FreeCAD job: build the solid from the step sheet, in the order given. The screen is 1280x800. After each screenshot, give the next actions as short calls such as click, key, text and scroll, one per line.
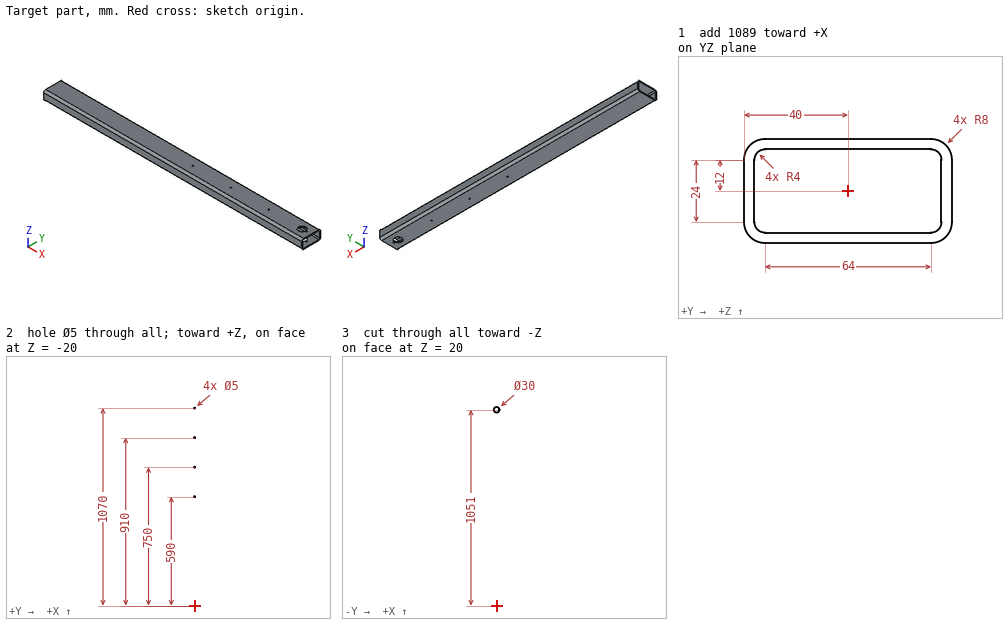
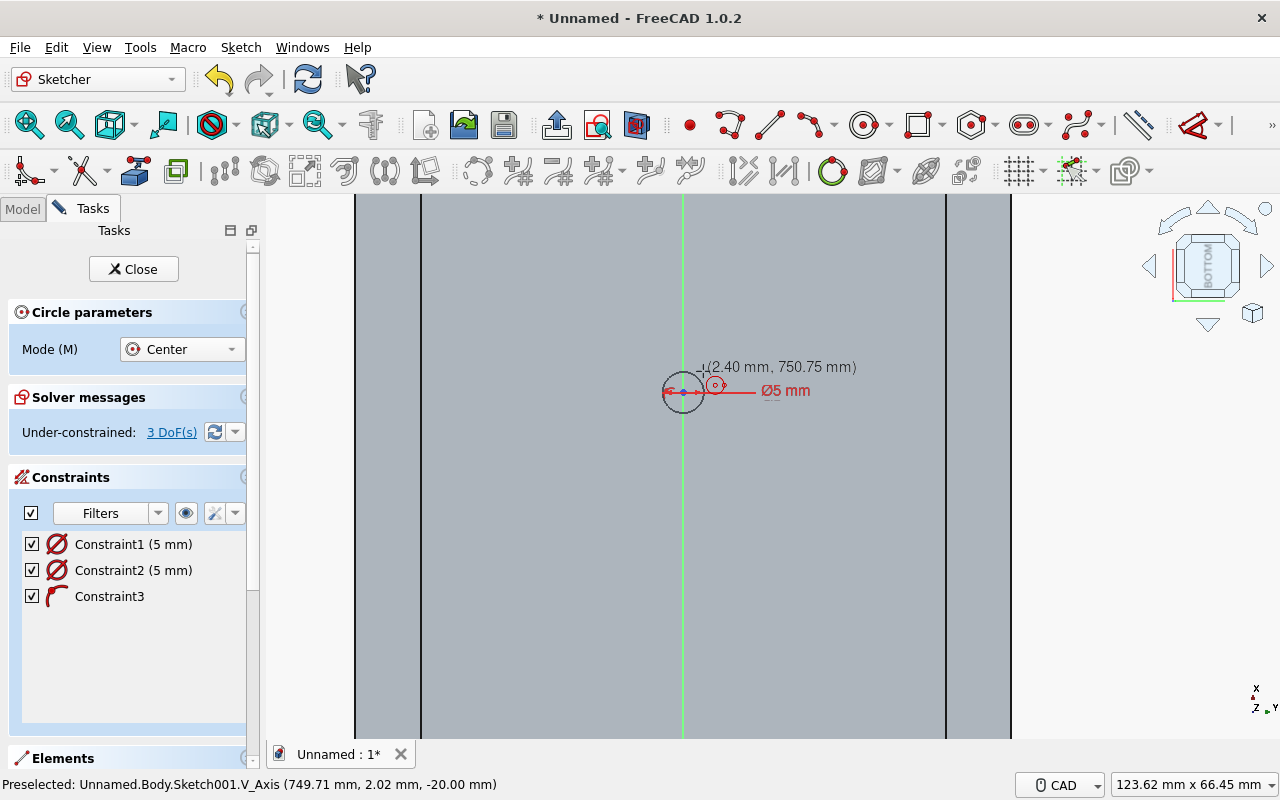
scroll(706, 379, down, 15)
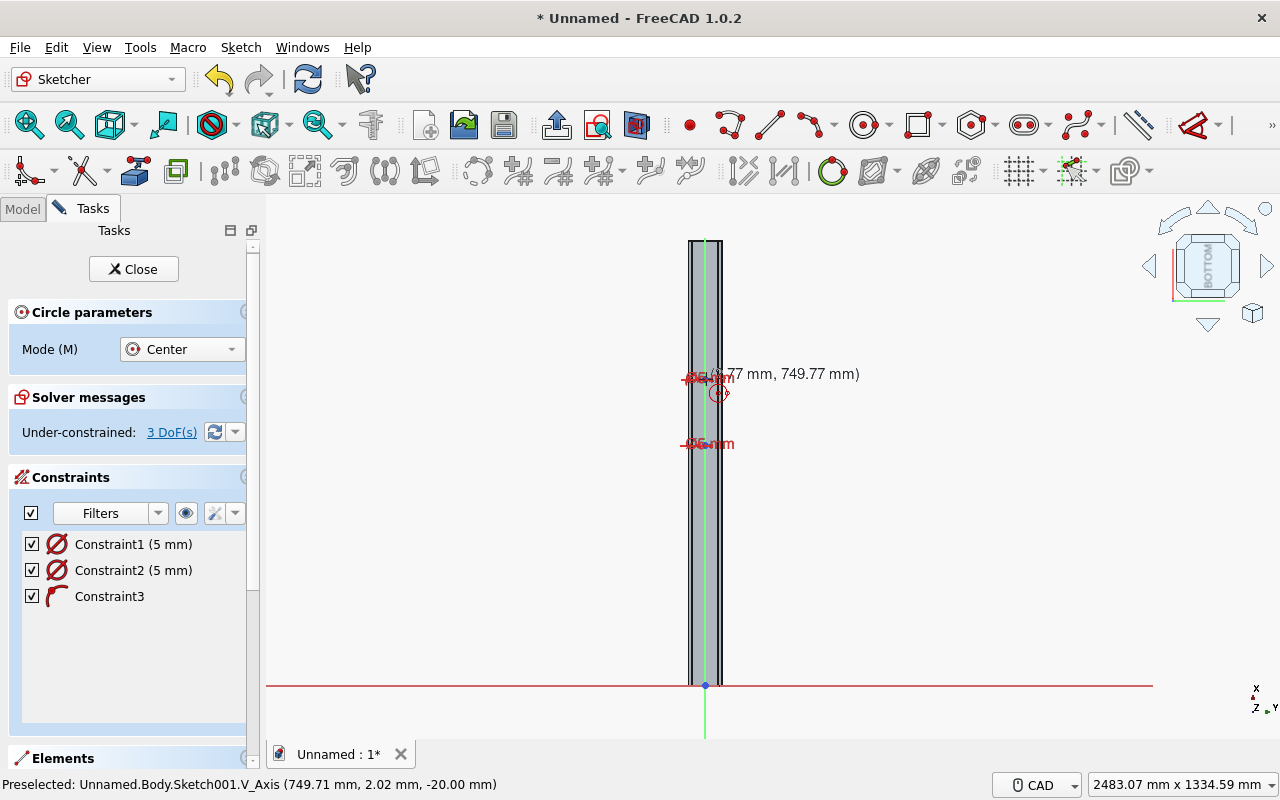
scroll(705, 314, up, 16)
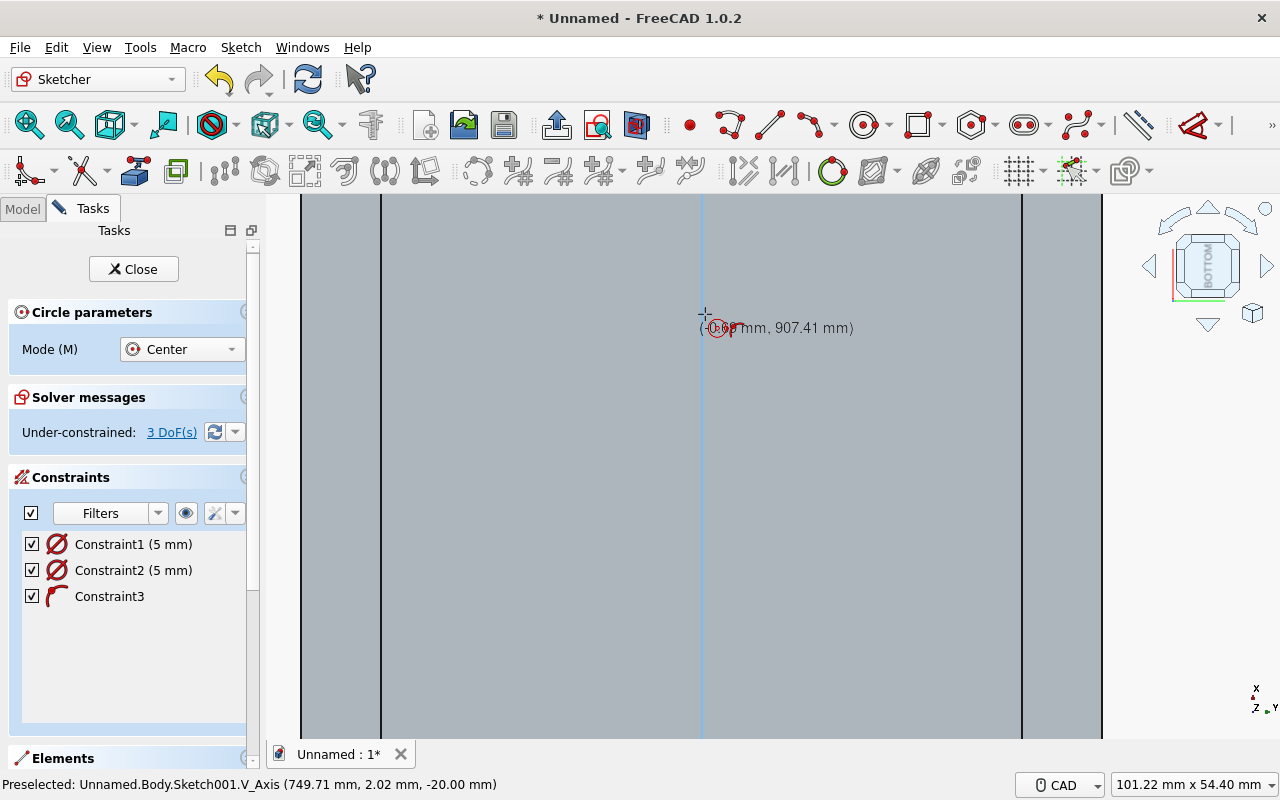
scroll(705, 314, down, 16)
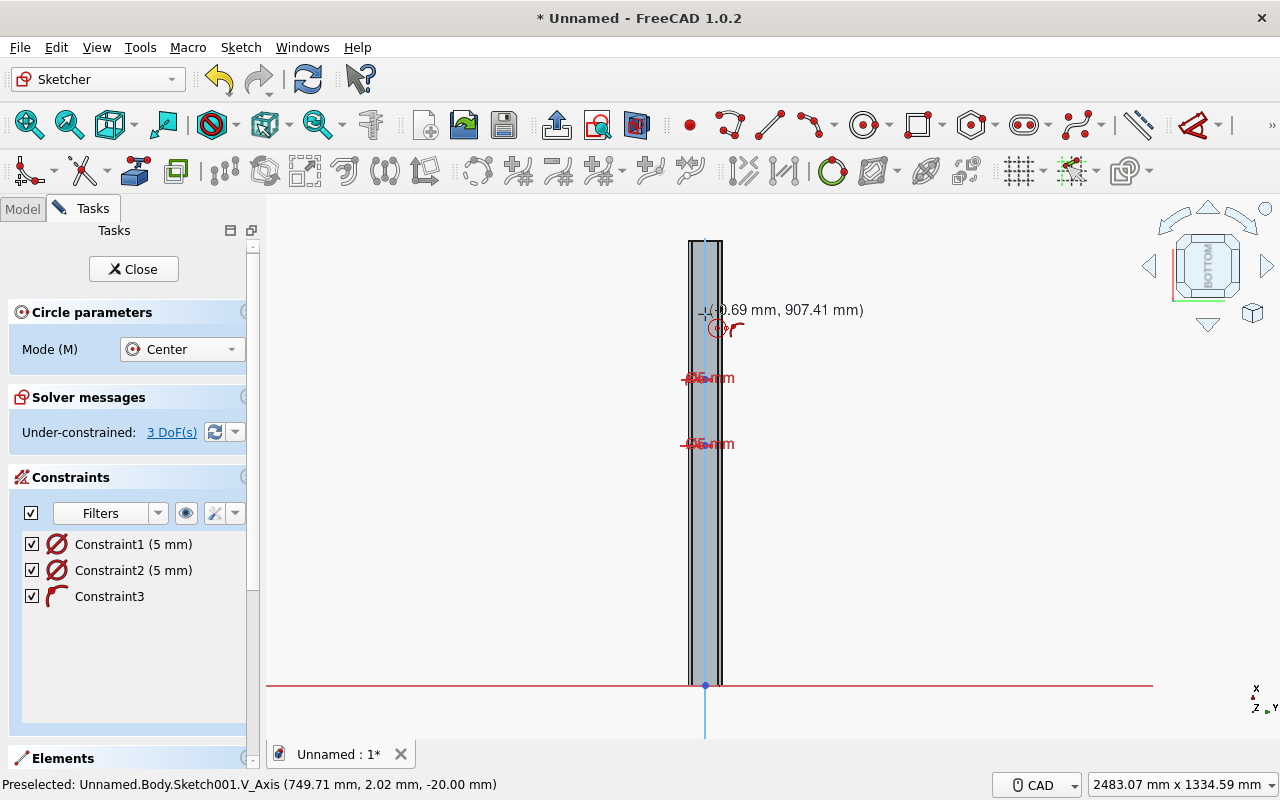
click(705, 314)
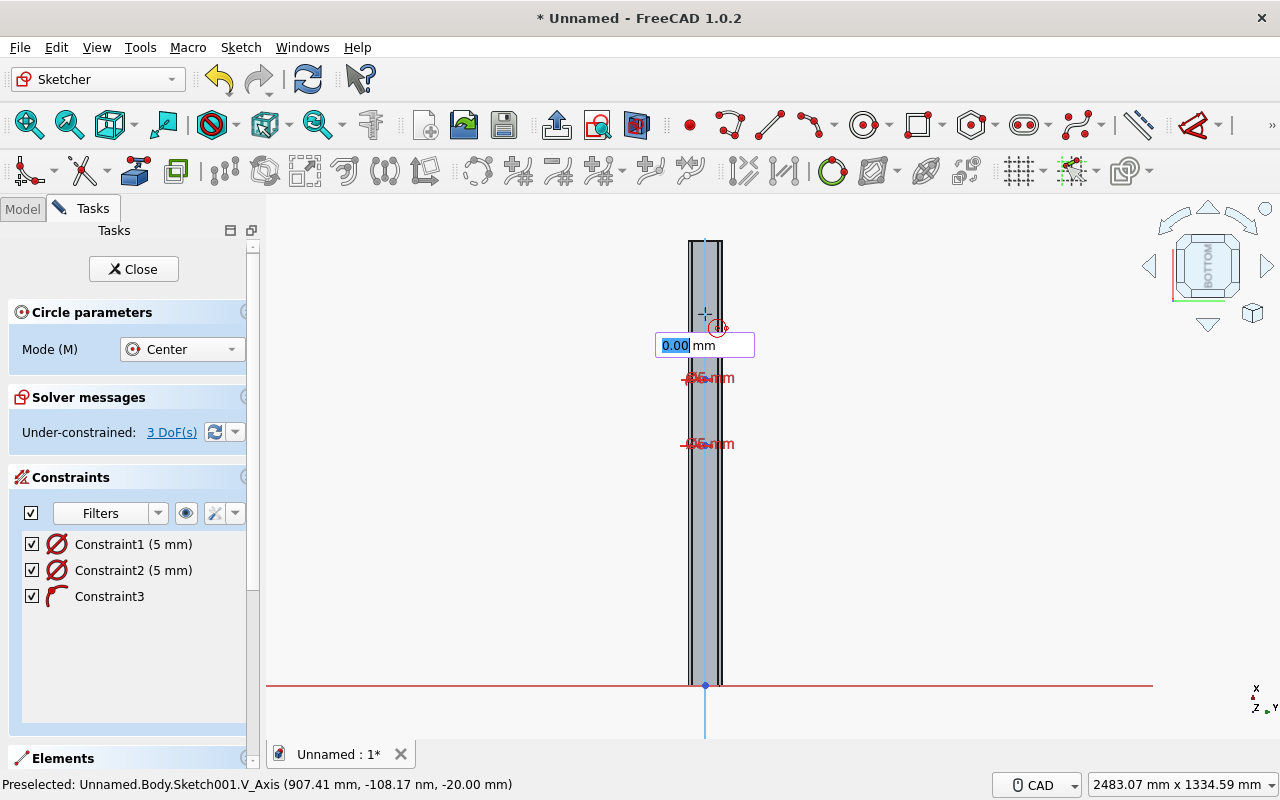
scroll(706, 314, up, 15)
move(703, 302)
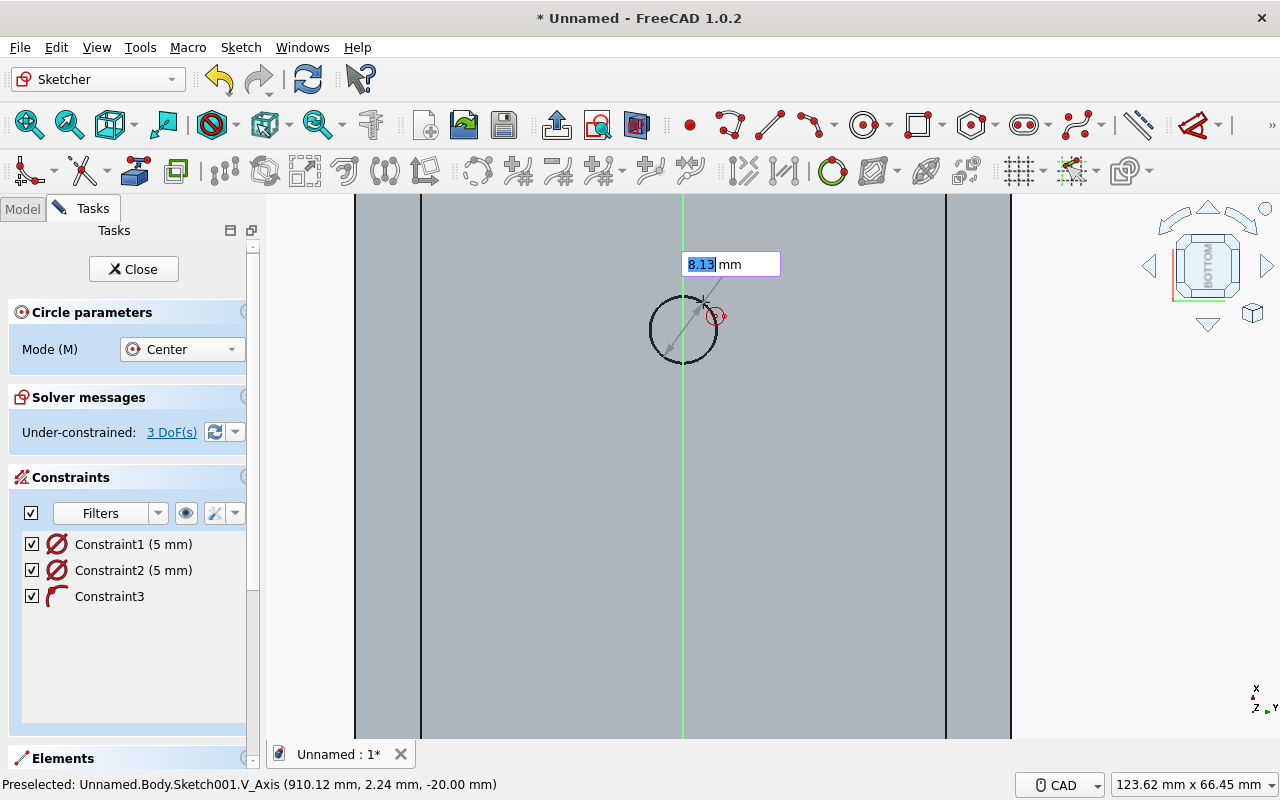
text(5)
key(Return)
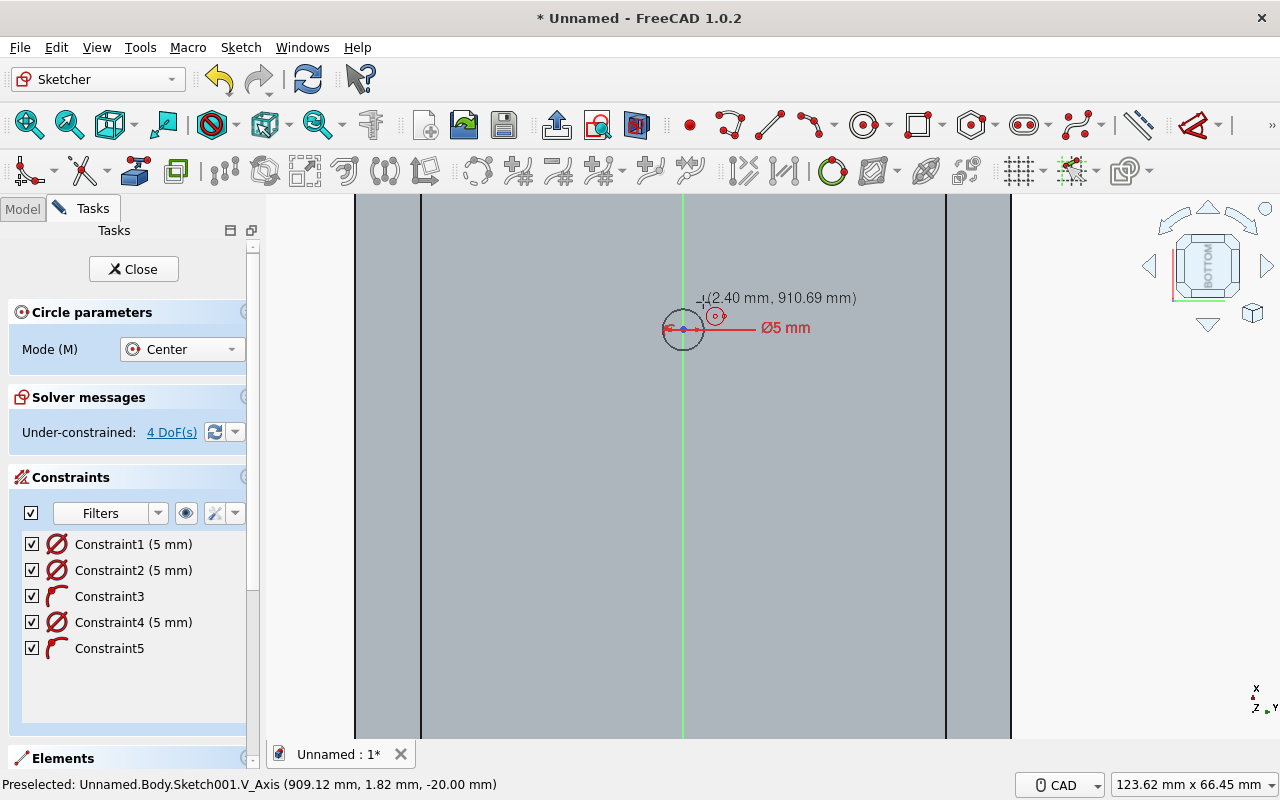
scroll(706, 314, down, 15)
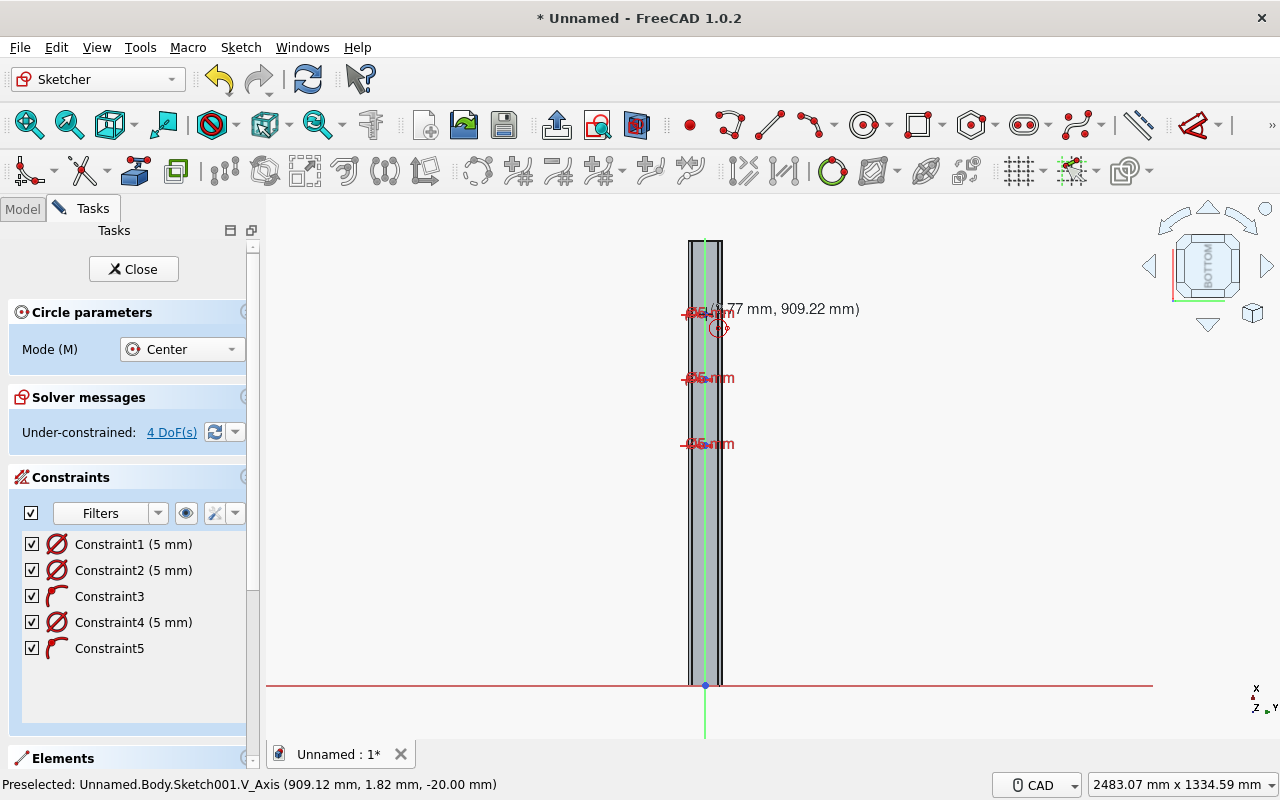
scroll(705, 249, up, 16)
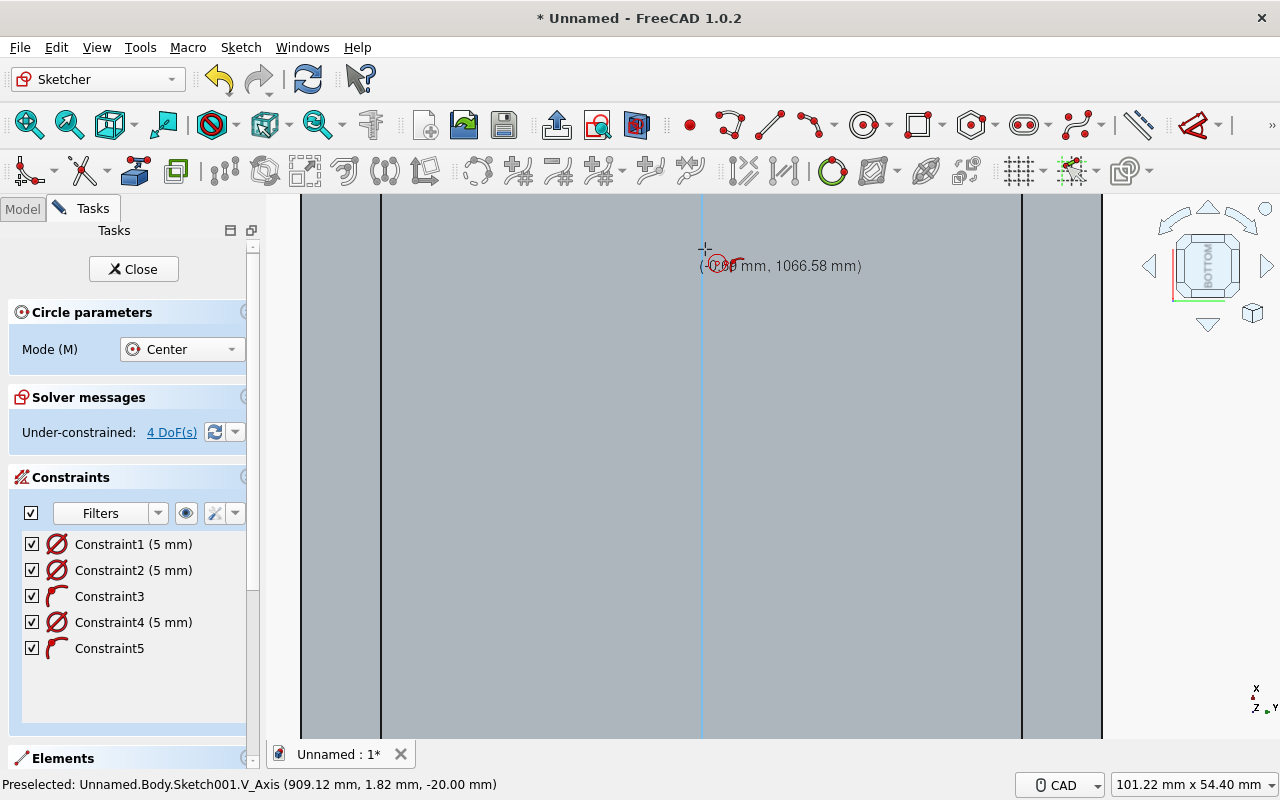
scroll(705, 249, down, 16)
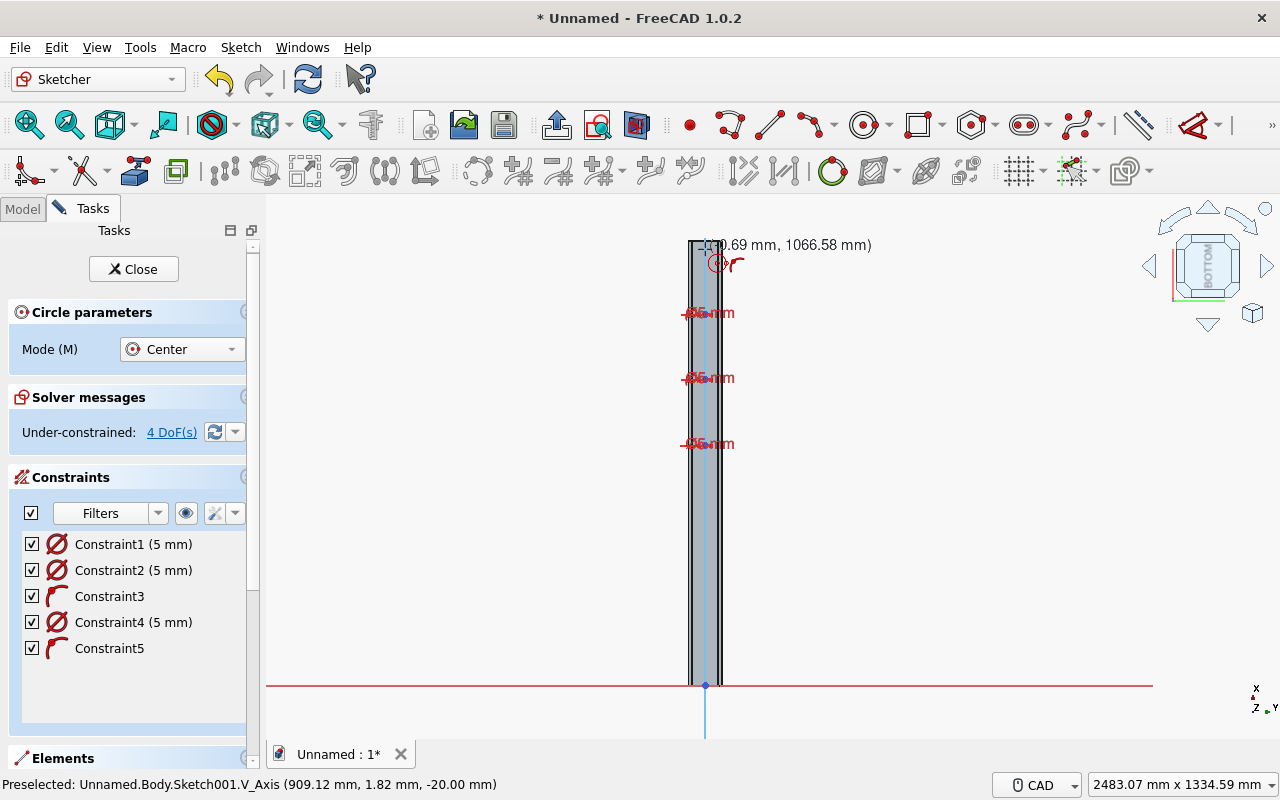
click(705, 249)